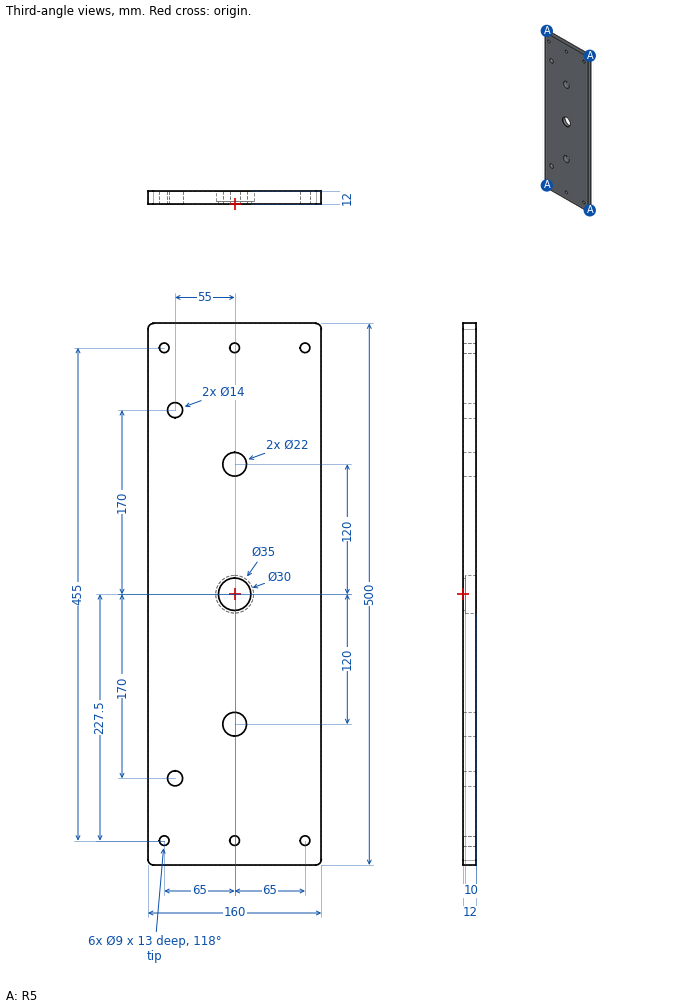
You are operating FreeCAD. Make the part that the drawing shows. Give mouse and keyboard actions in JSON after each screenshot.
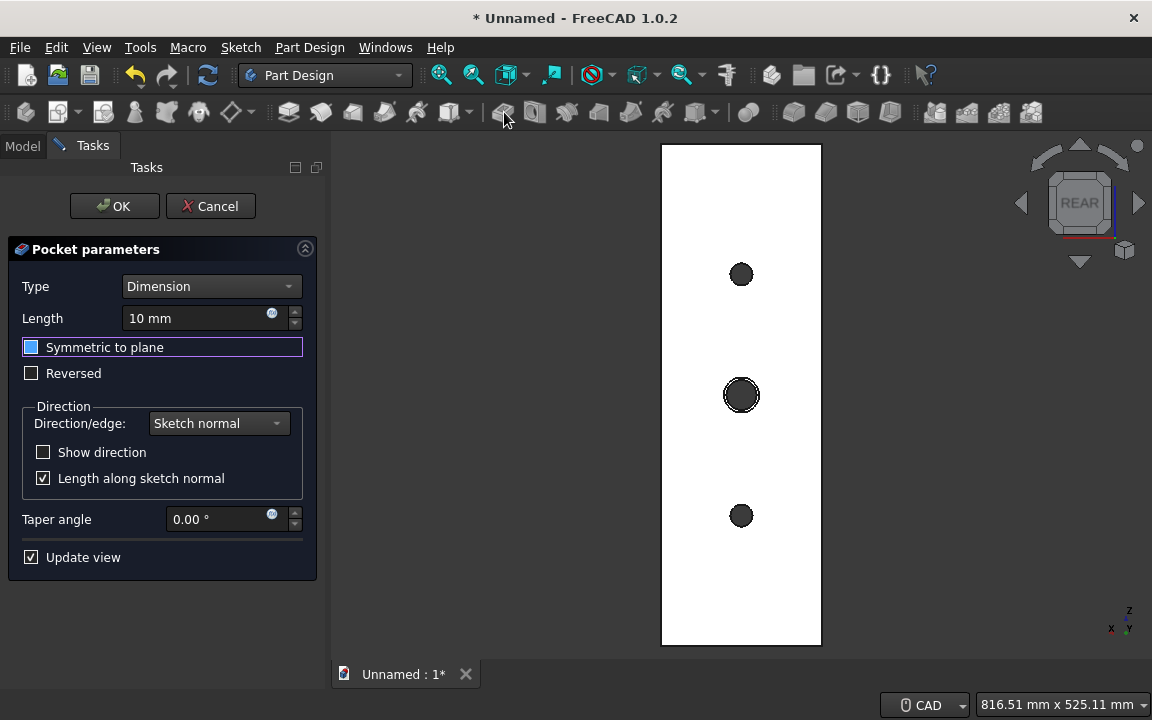
{"action": "left_click", "coordinate": [115, 206]}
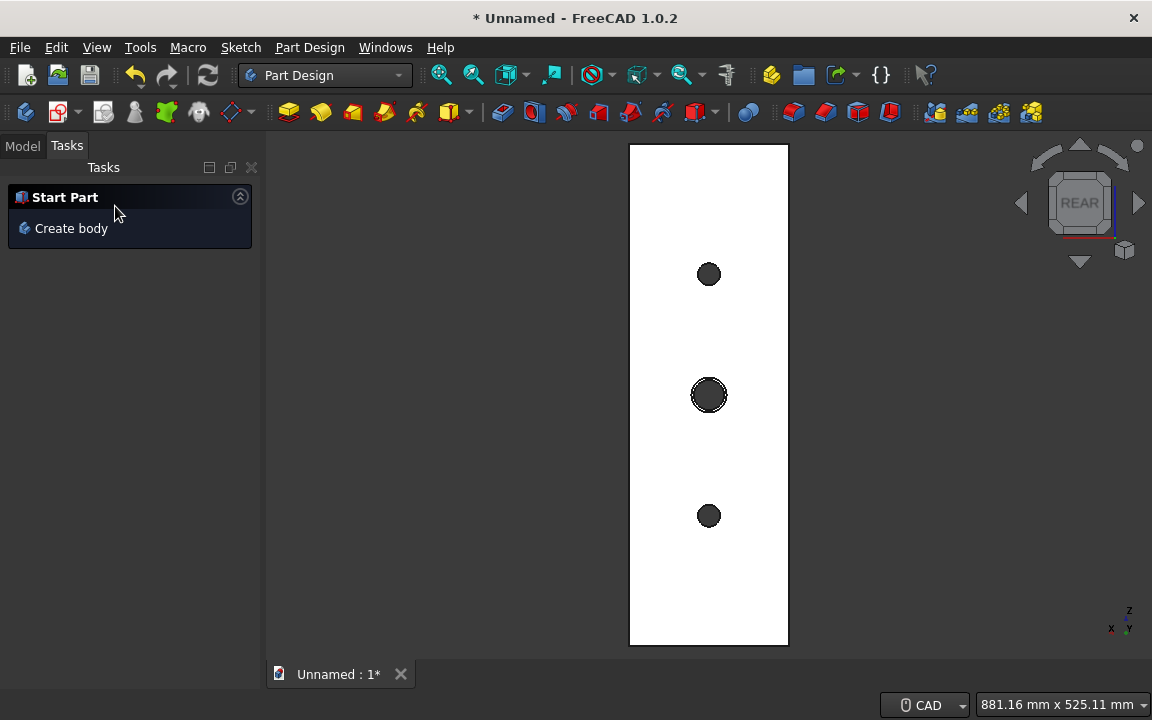
{"action": "left_click", "coordinate": [686, 466]}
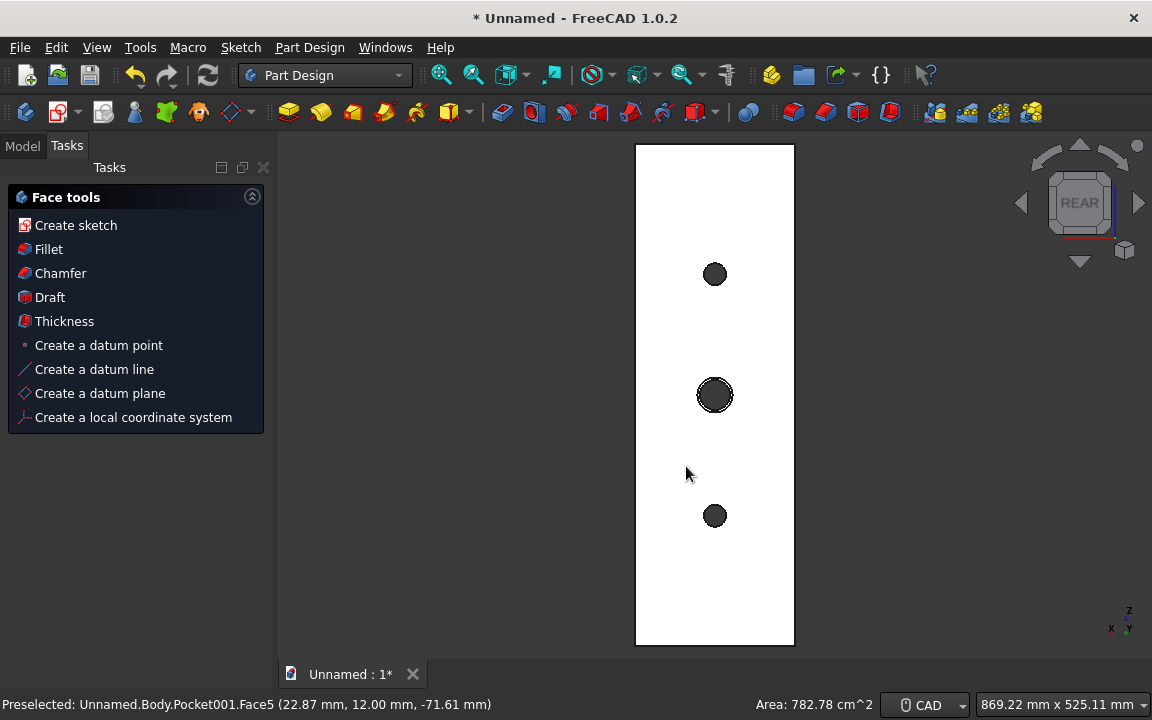
{"action": "left_click", "coordinate": [58, 112]}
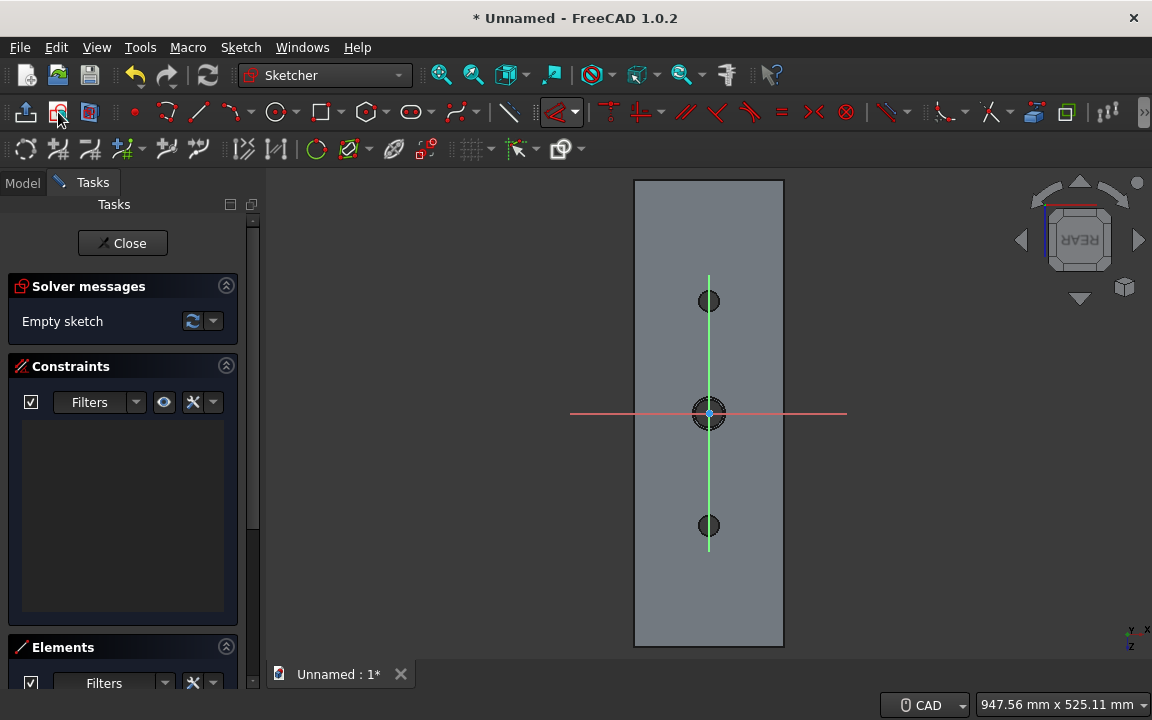
{"action": "scroll", "coordinate": [501, 414], "scroll_direction": "down", "scroll_amount": 2}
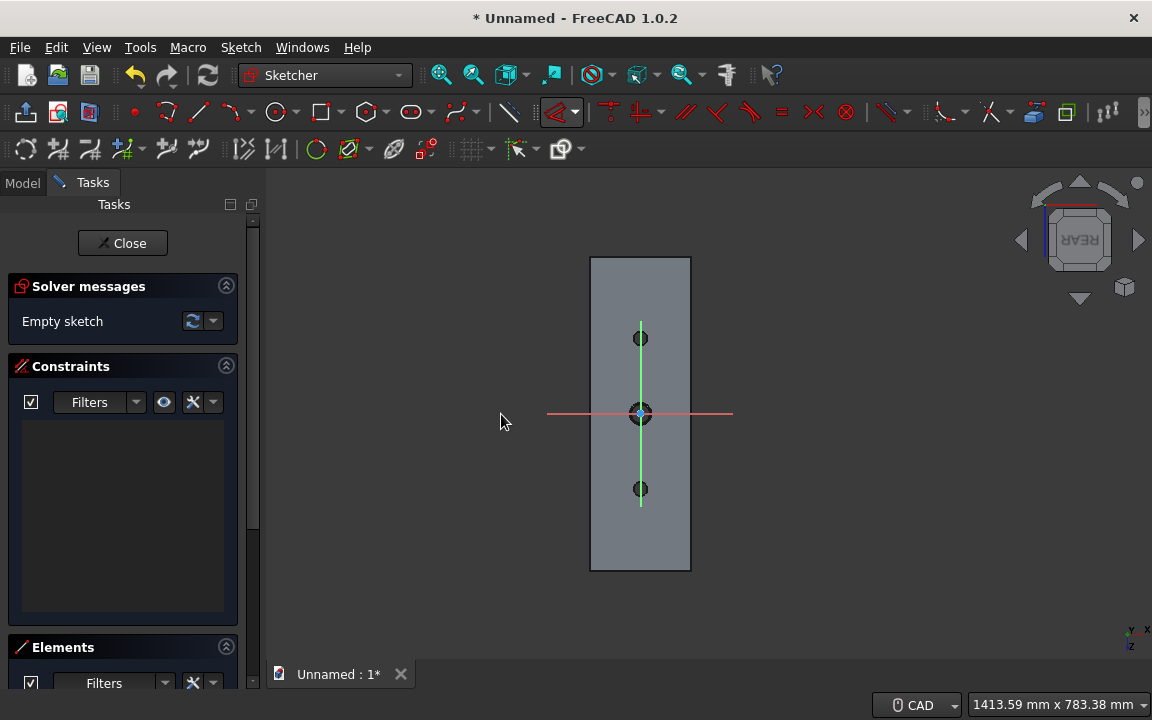
{"action": "left_click", "coordinate": [276, 112]}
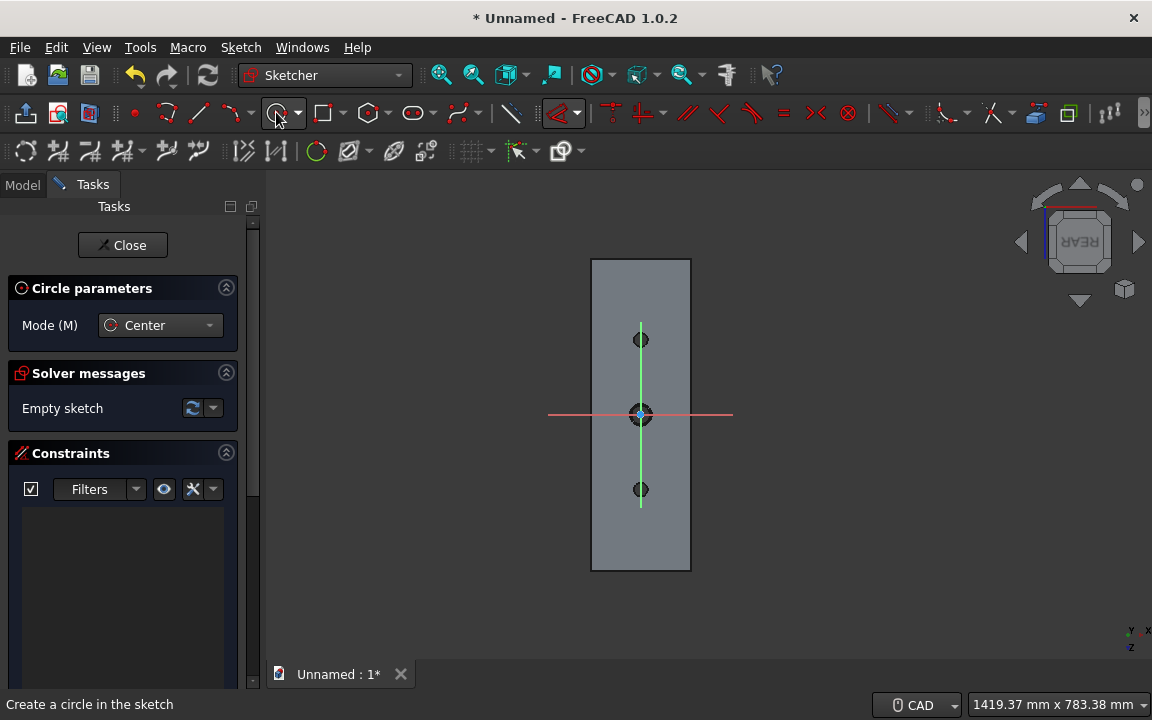
{"action": "scroll", "coordinate": [600, 273], "scroll_direction": "up", "scroll_amount": 11}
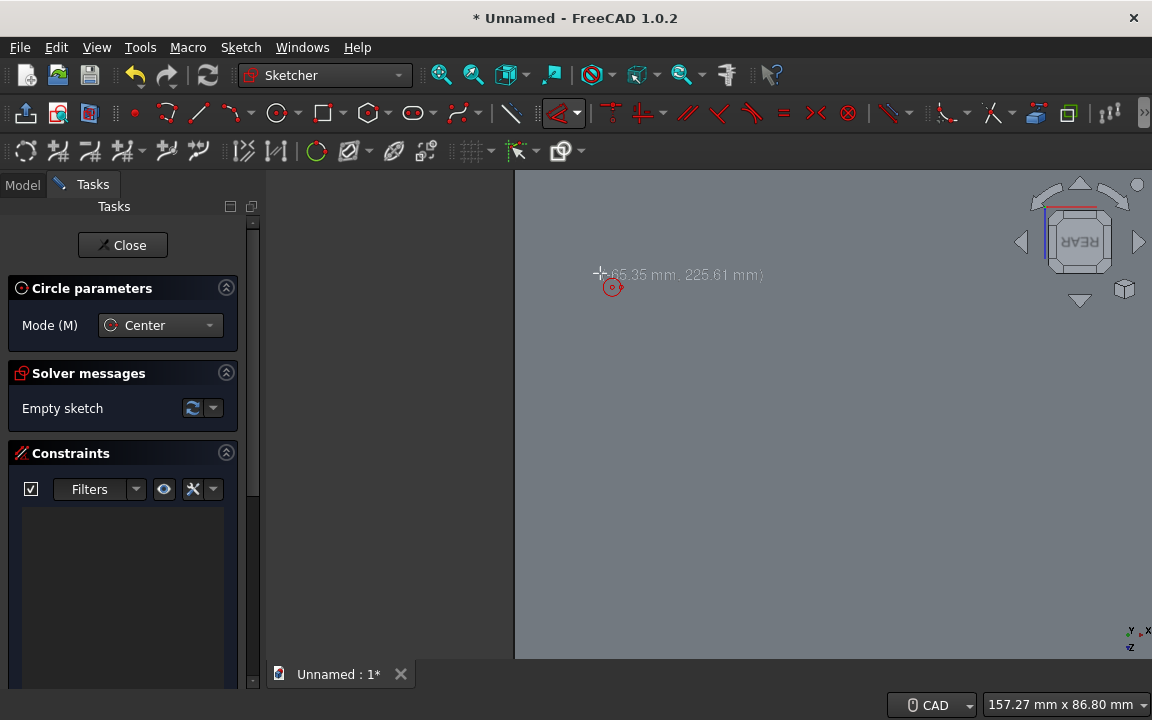
{"action": "scroll", "coordinate": [600, 273], "scroll_direction": "down", "scroll_amount": 11}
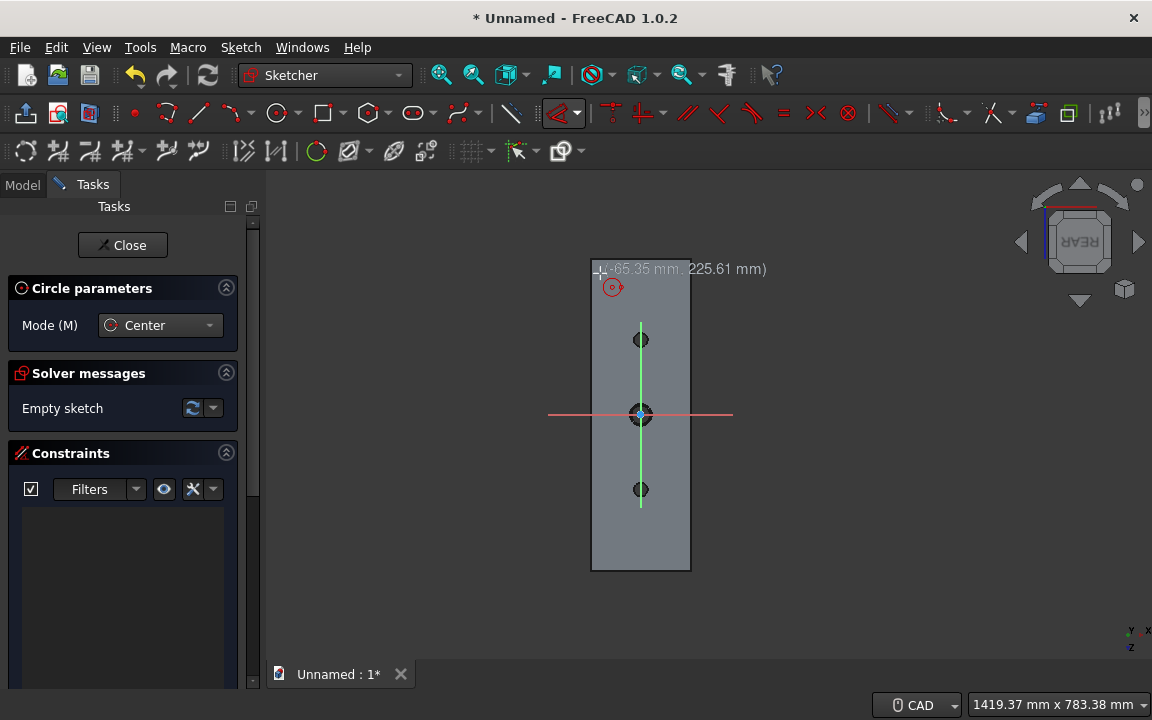
{"action": "left_click", "coordinate": [600, 273]}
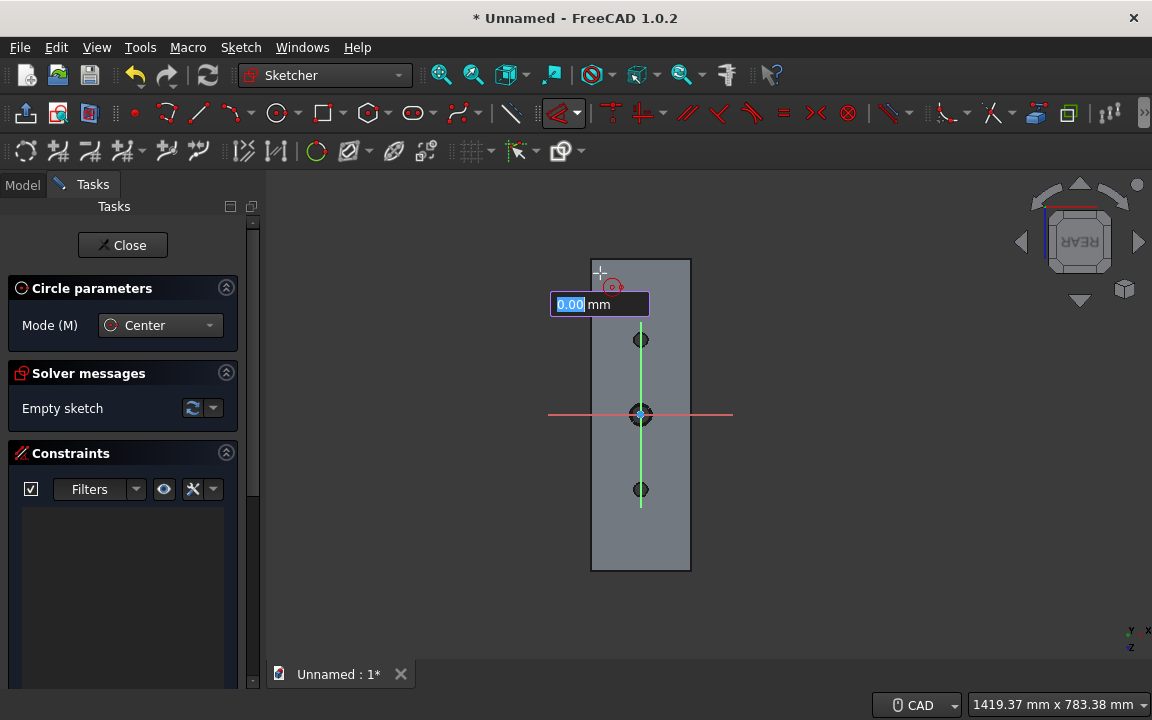
{"action": "scroll", "coordinate": [602, 271], "scroll_direction": "up", "scroll_amount": 9}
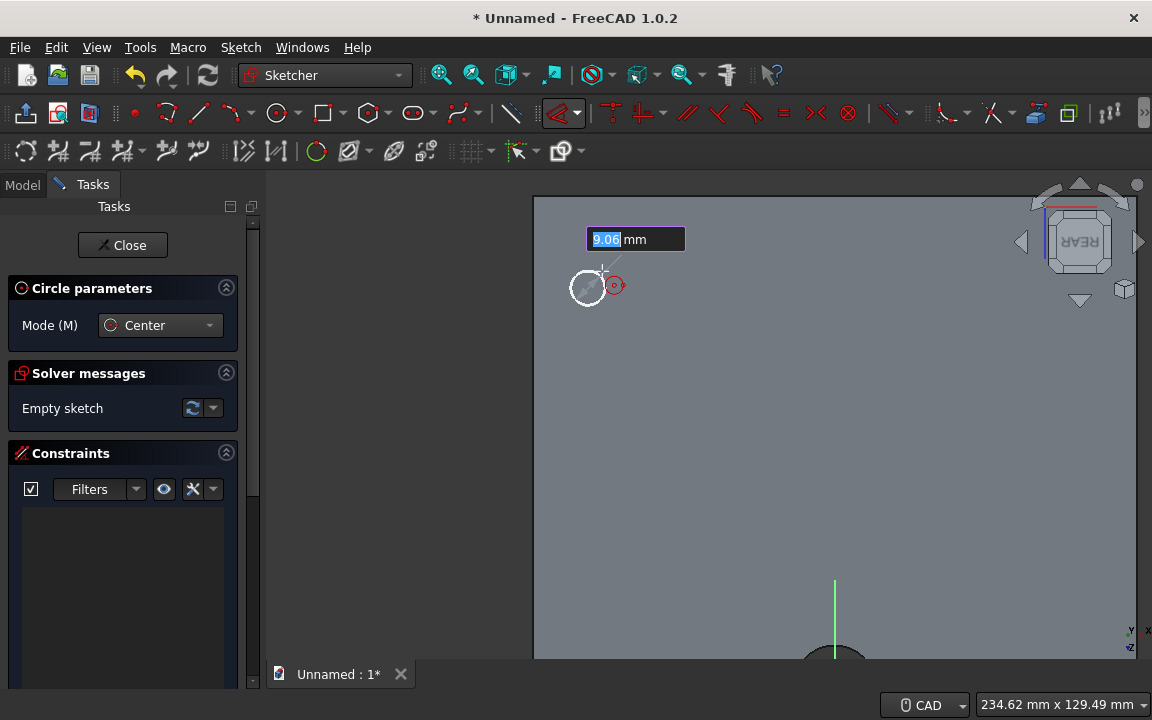
{"action": "left_click", "coordinate": [601, 269]}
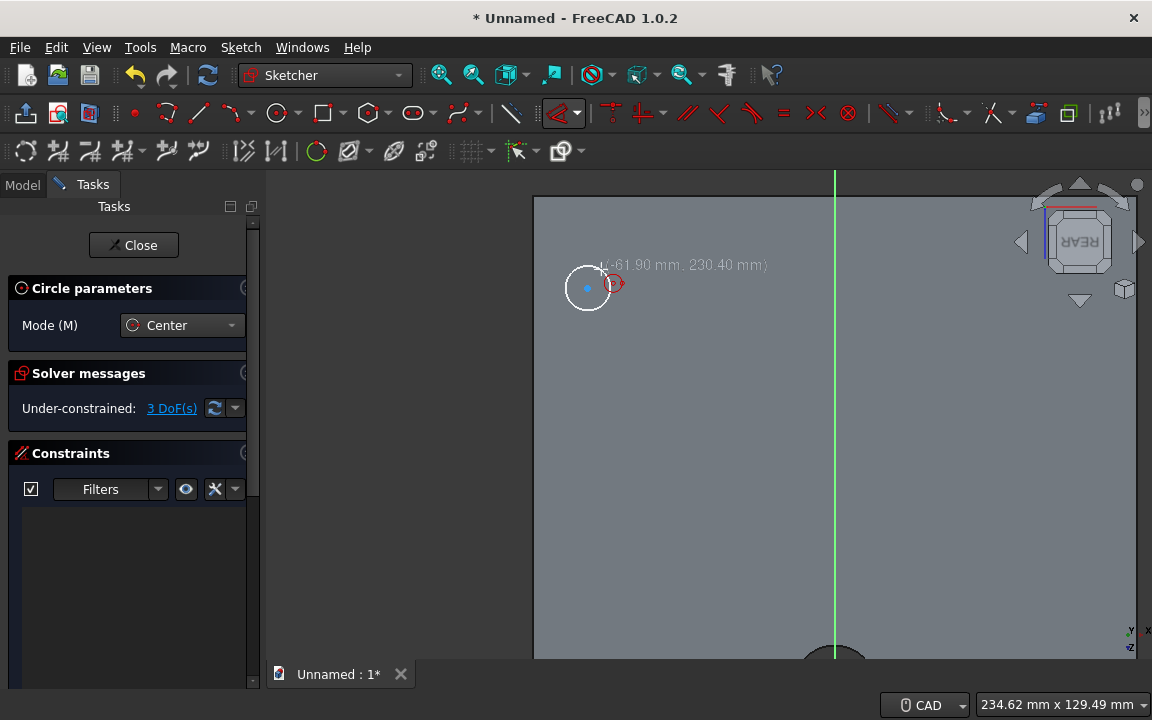
{"action": "scroll", "coordinate": [835, 281], "scroll_direction": "up", "scroll_amount": 2}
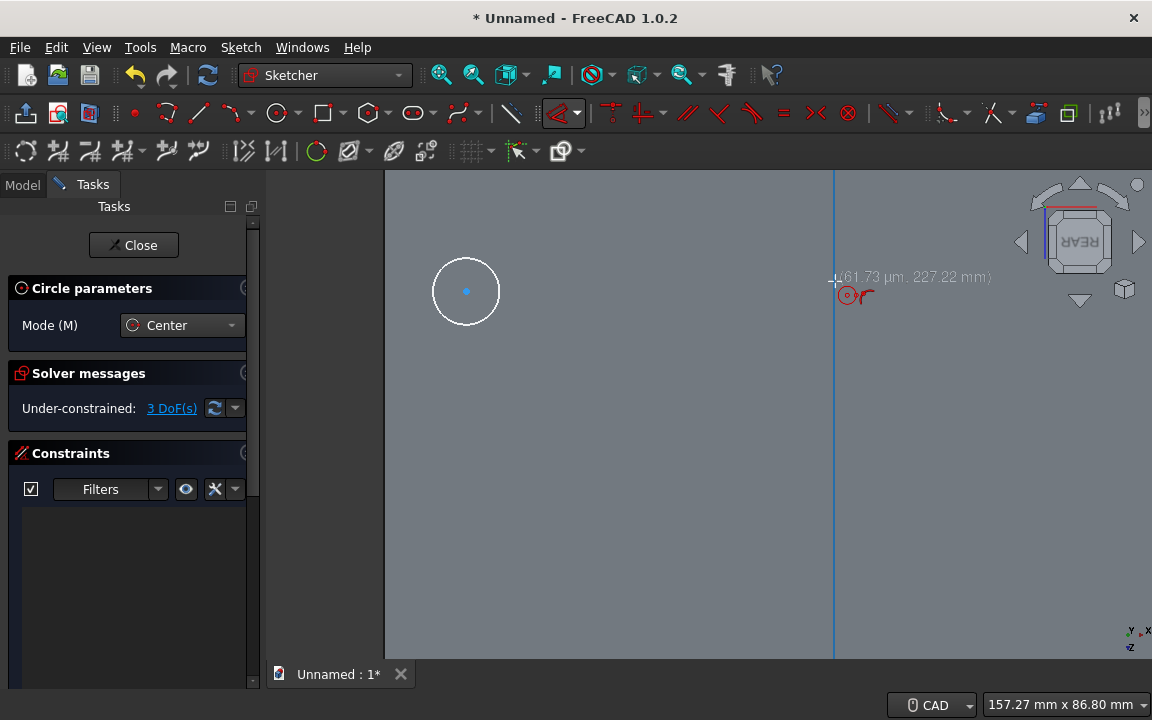
{"action": "scroll", "coordinate": [616, 271], "scroll_direction": "down", "scroll_amount": 11}